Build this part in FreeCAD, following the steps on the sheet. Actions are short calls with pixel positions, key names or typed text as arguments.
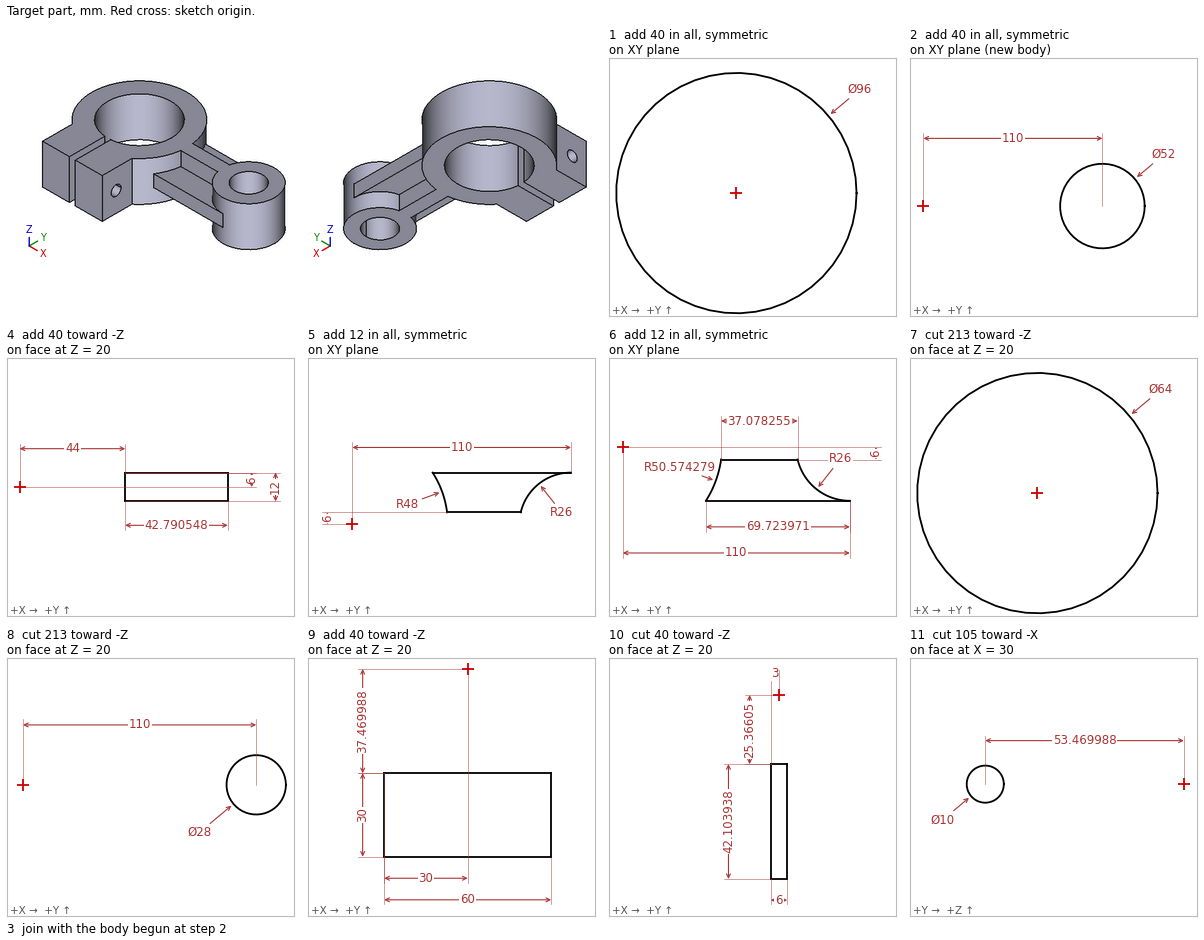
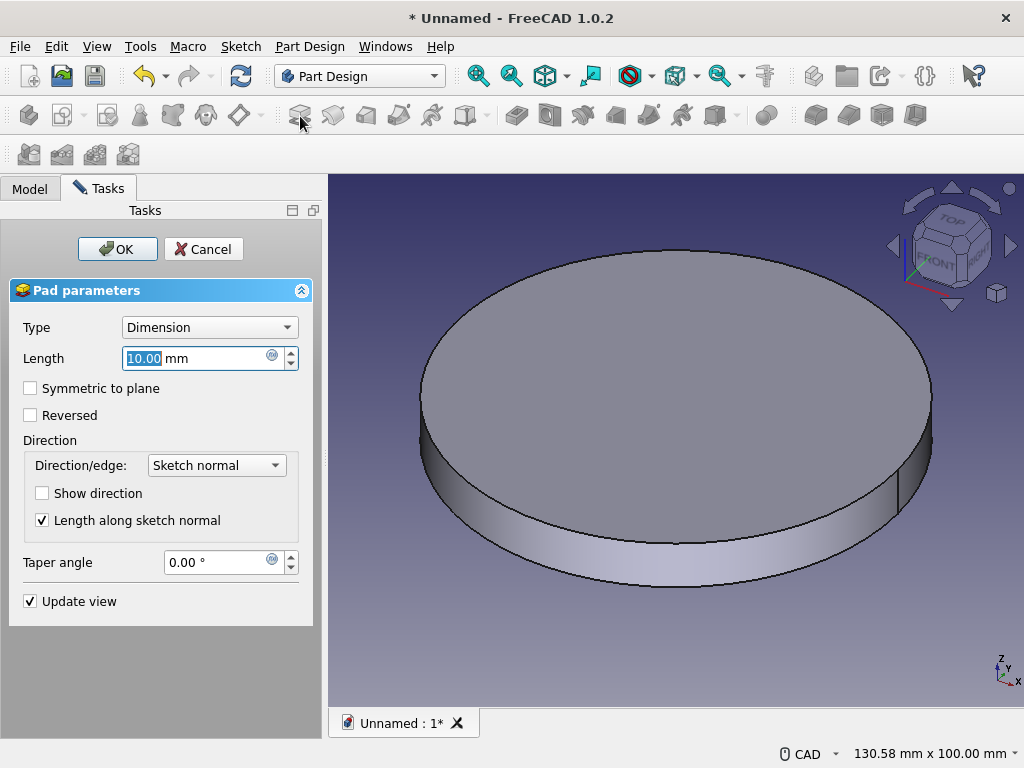
text(40)
key(Tab)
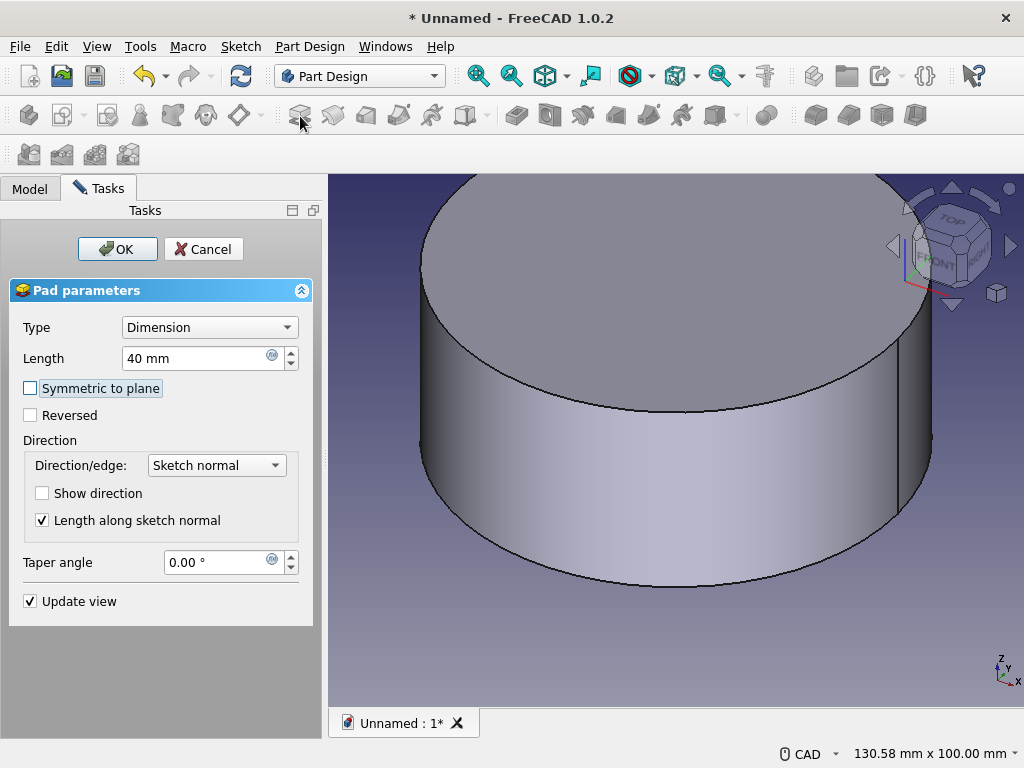
click(31, 388)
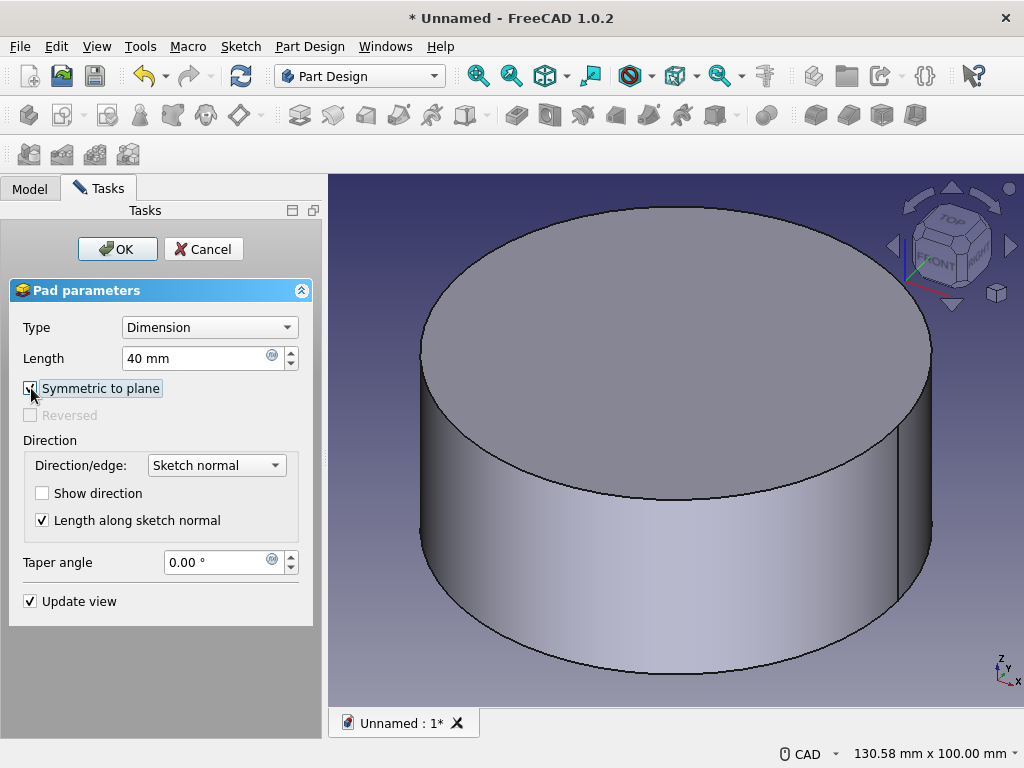
click(118, 249)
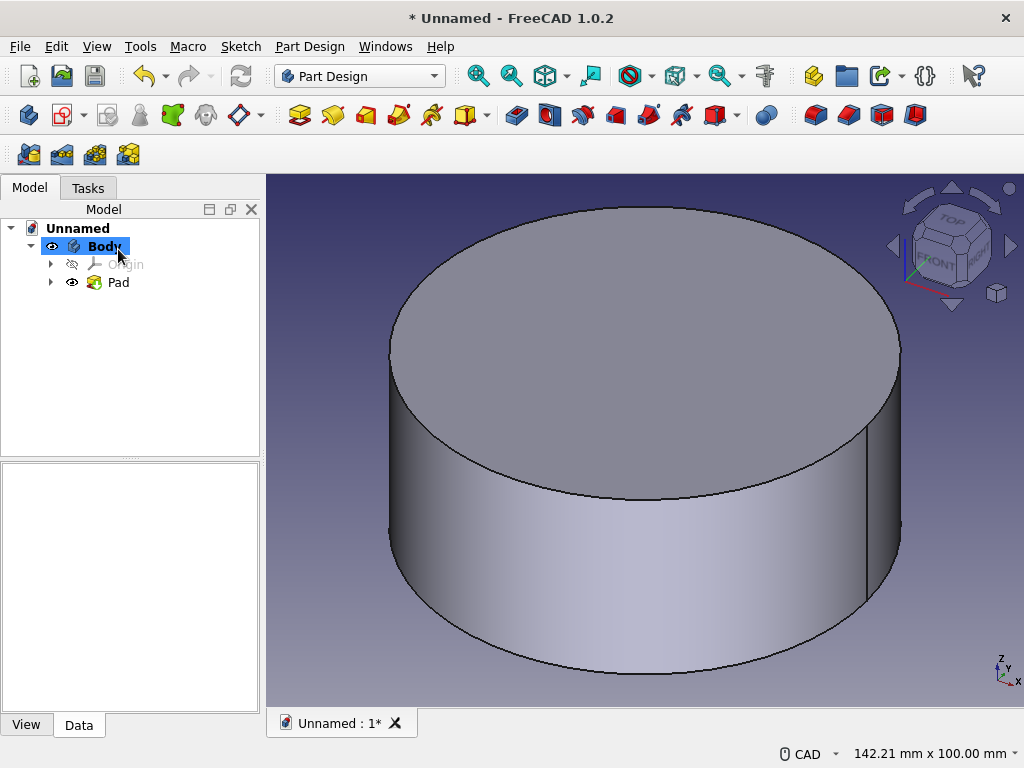
click(479, 76)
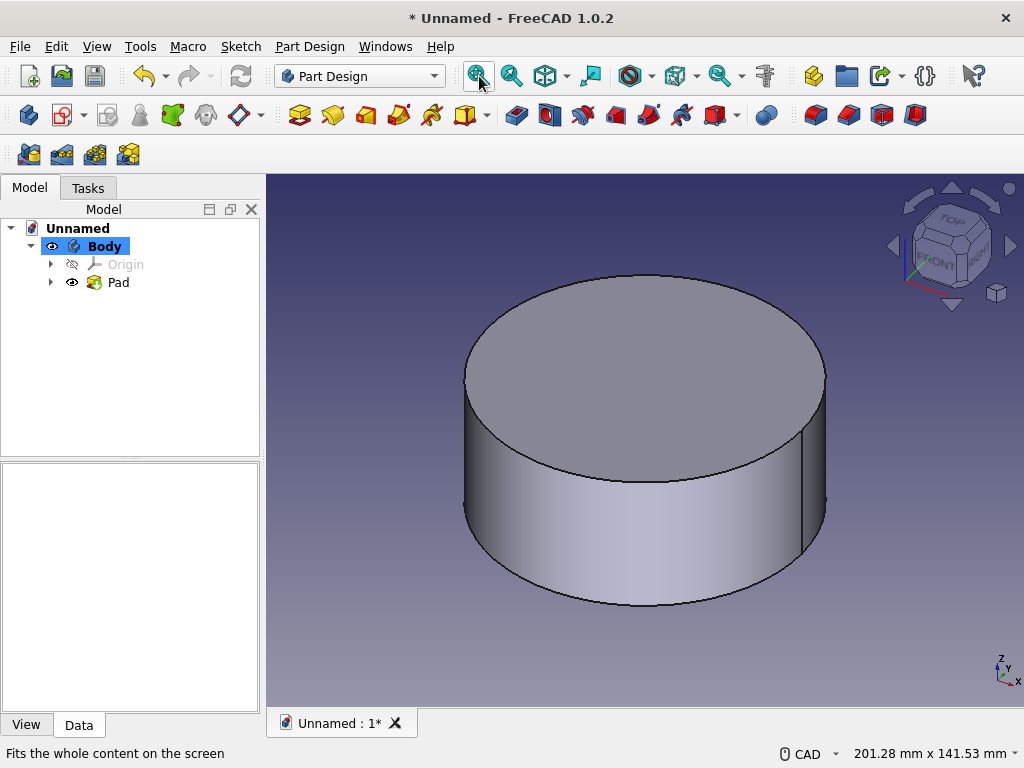
click(29, 116)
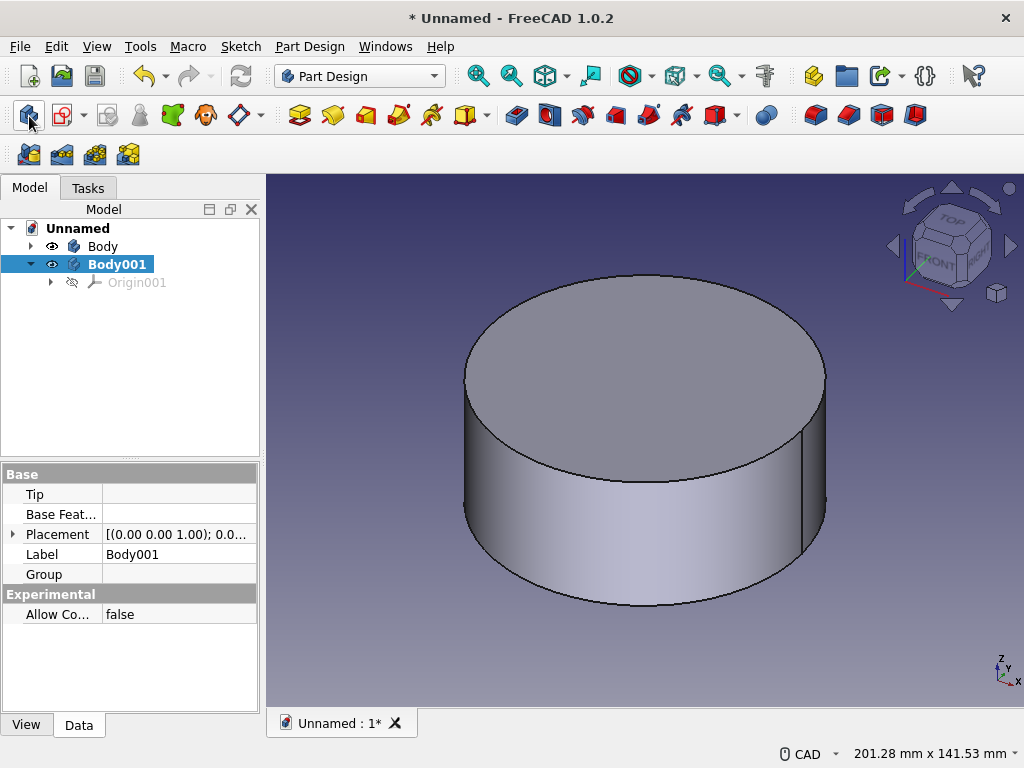
click(306, 667)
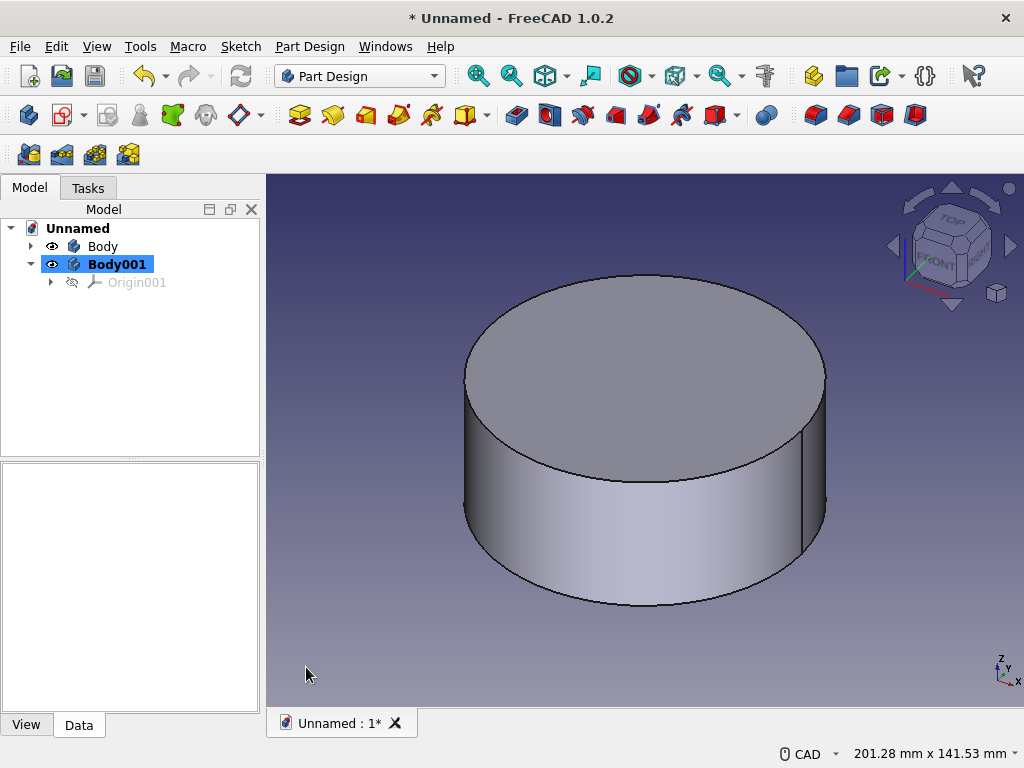
click(62, 116)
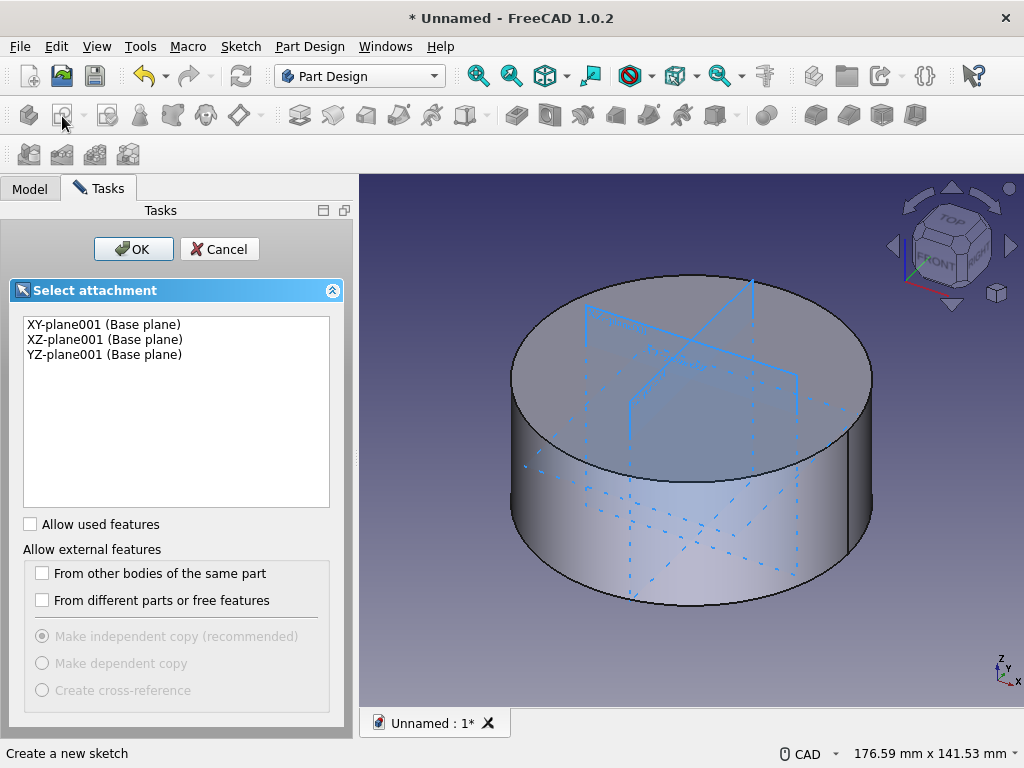
click(84, 324)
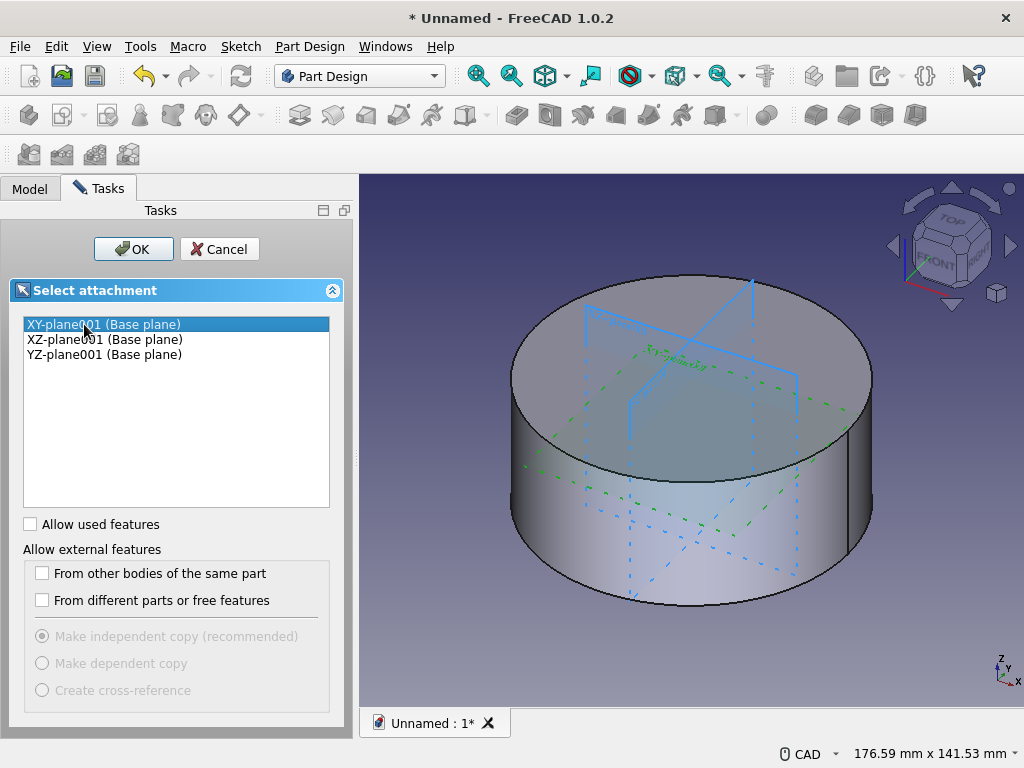
click(134, 249)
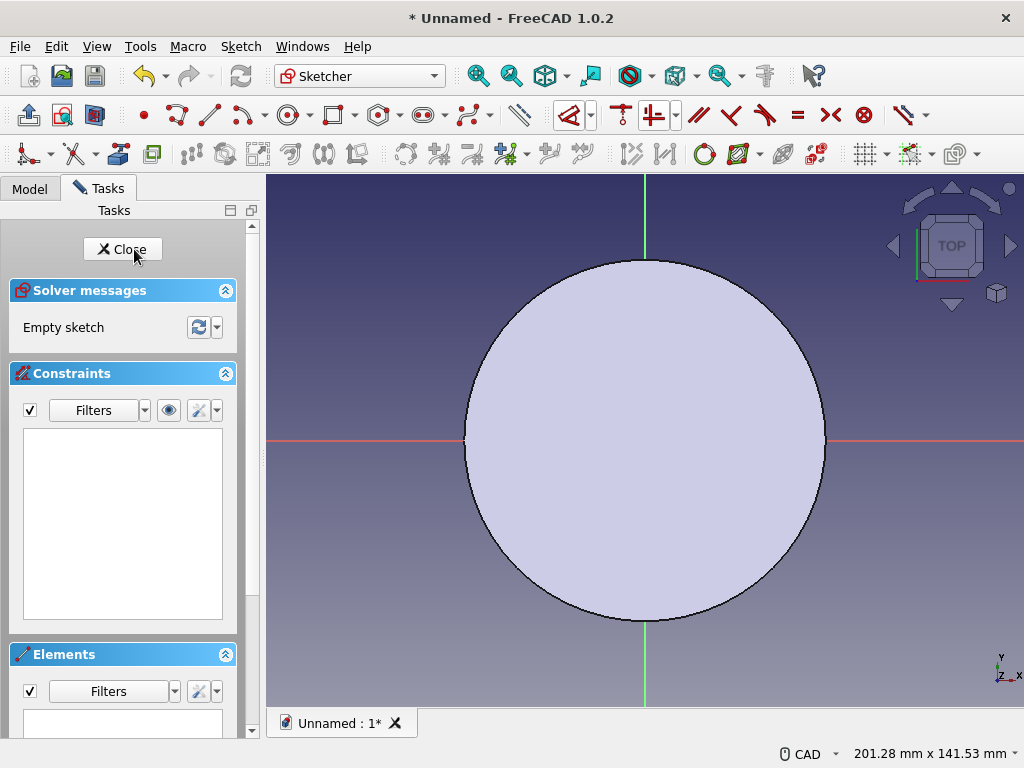
scroll(576, 440, down, 5)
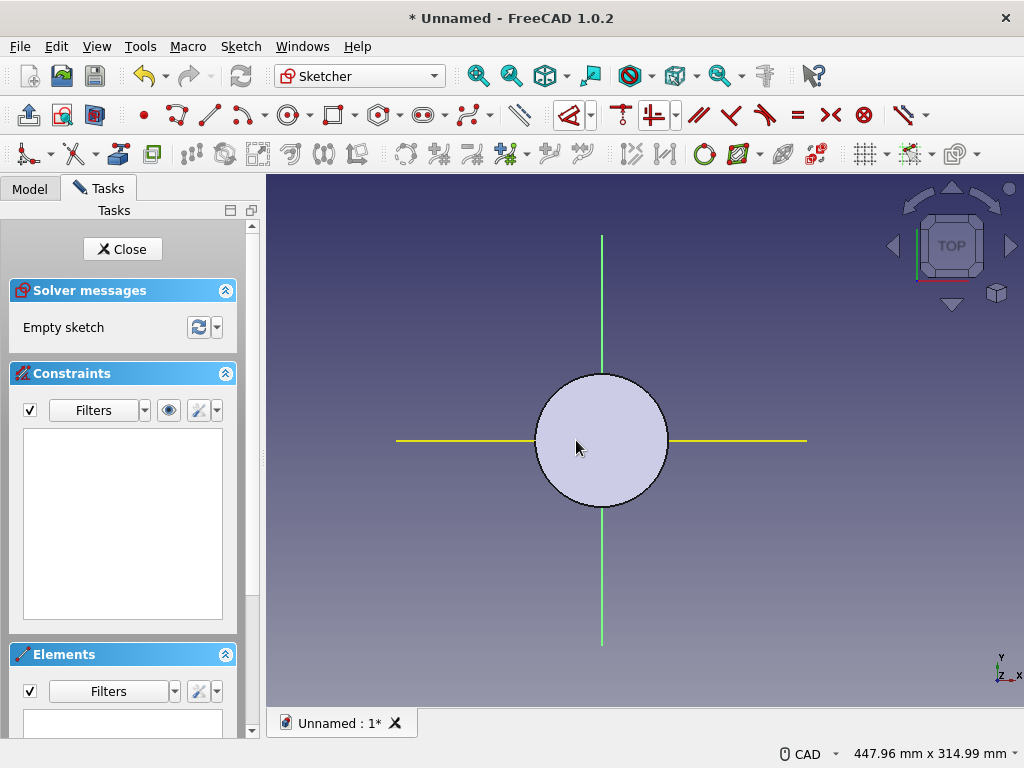
scroll(799, 440, up, 8)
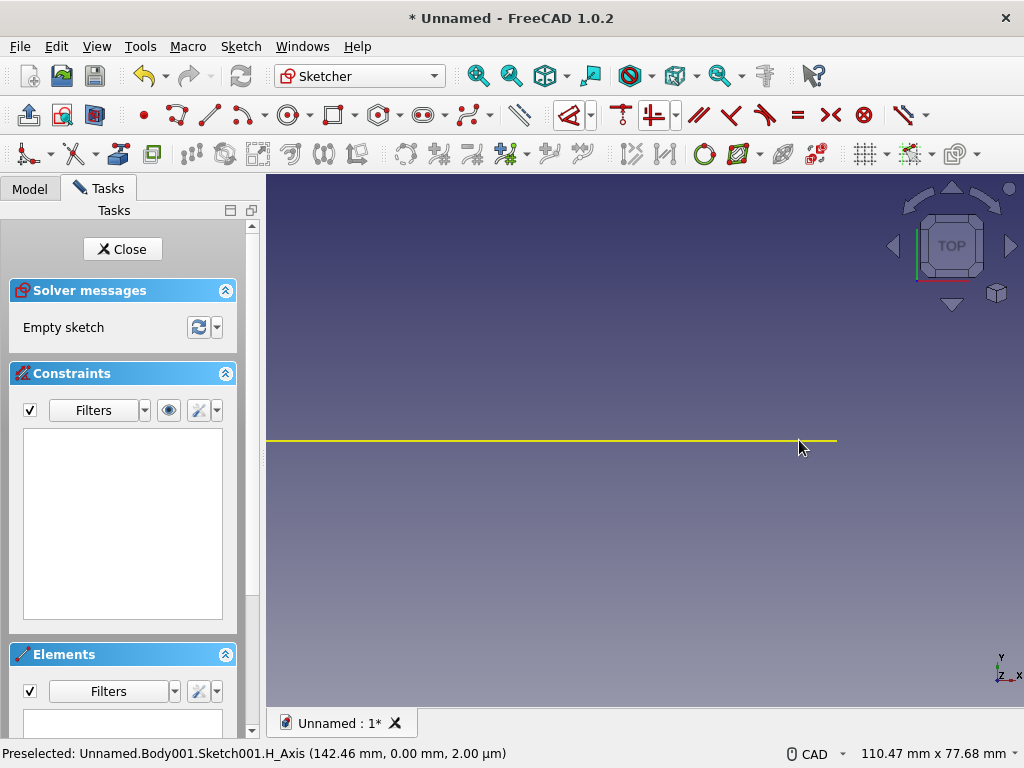
click(288, 116)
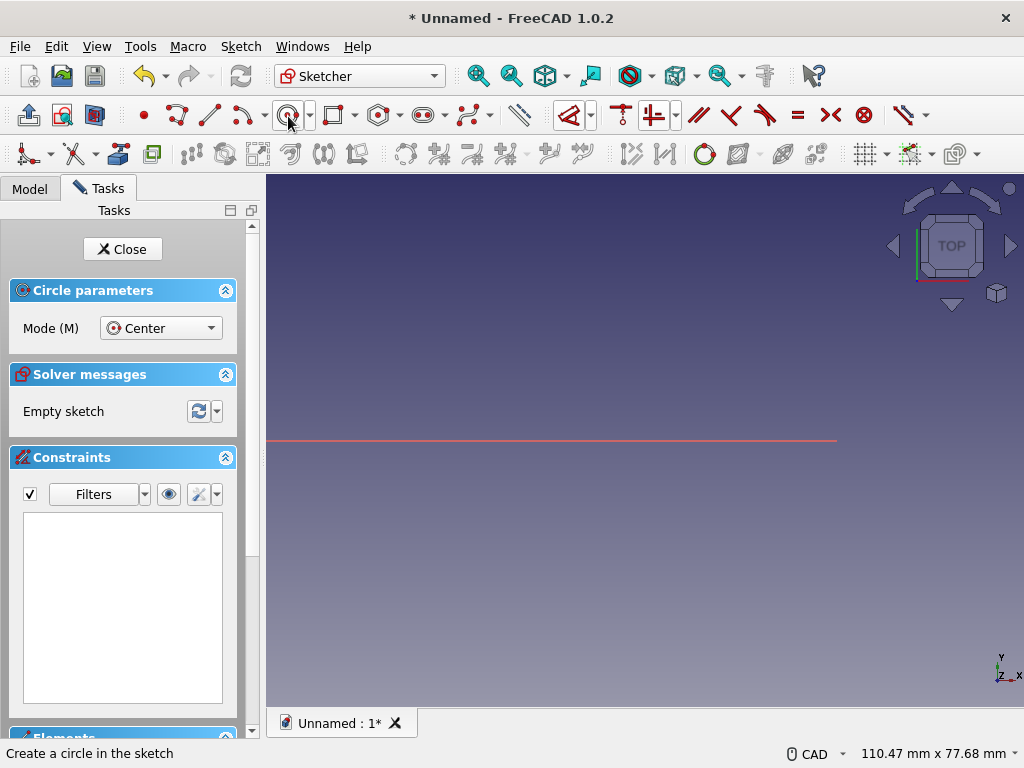
click(574, 440)
click(700, 314)
key(Escape)